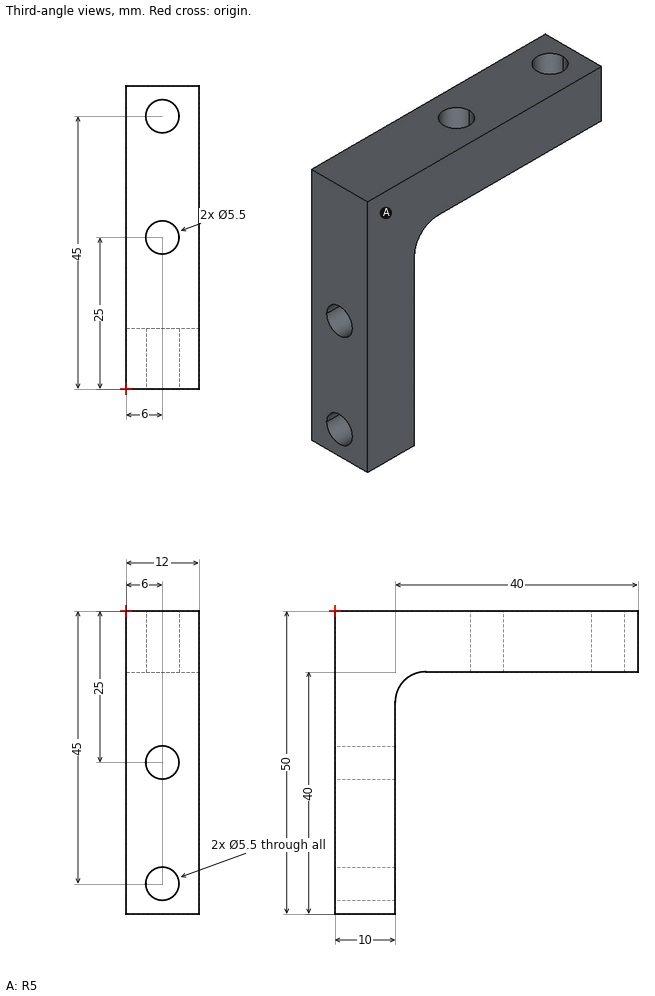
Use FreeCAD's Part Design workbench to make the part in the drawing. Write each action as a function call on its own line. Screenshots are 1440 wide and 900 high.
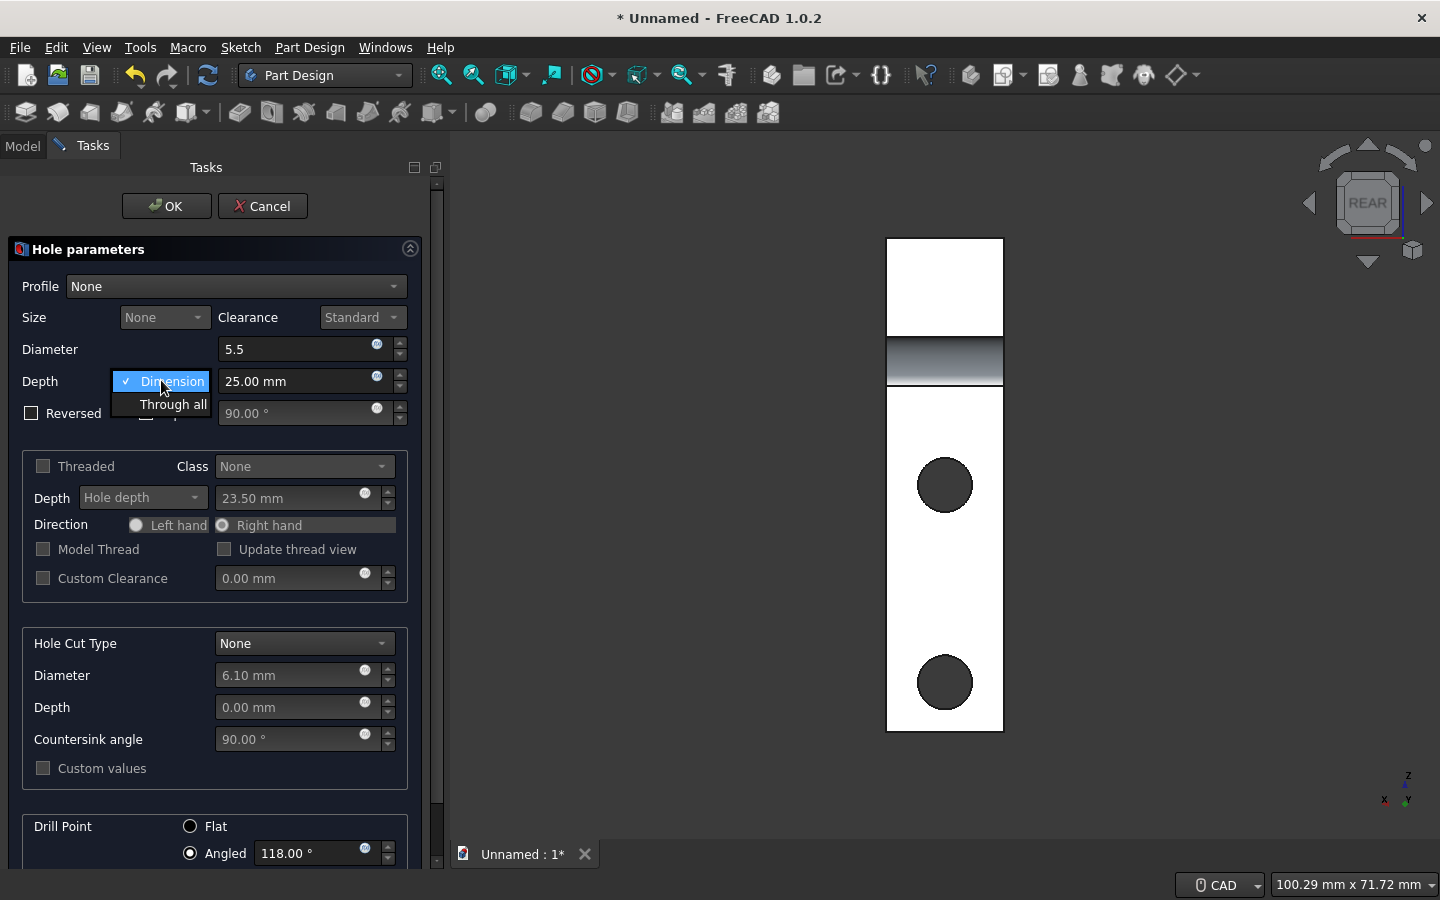
click(160, 404)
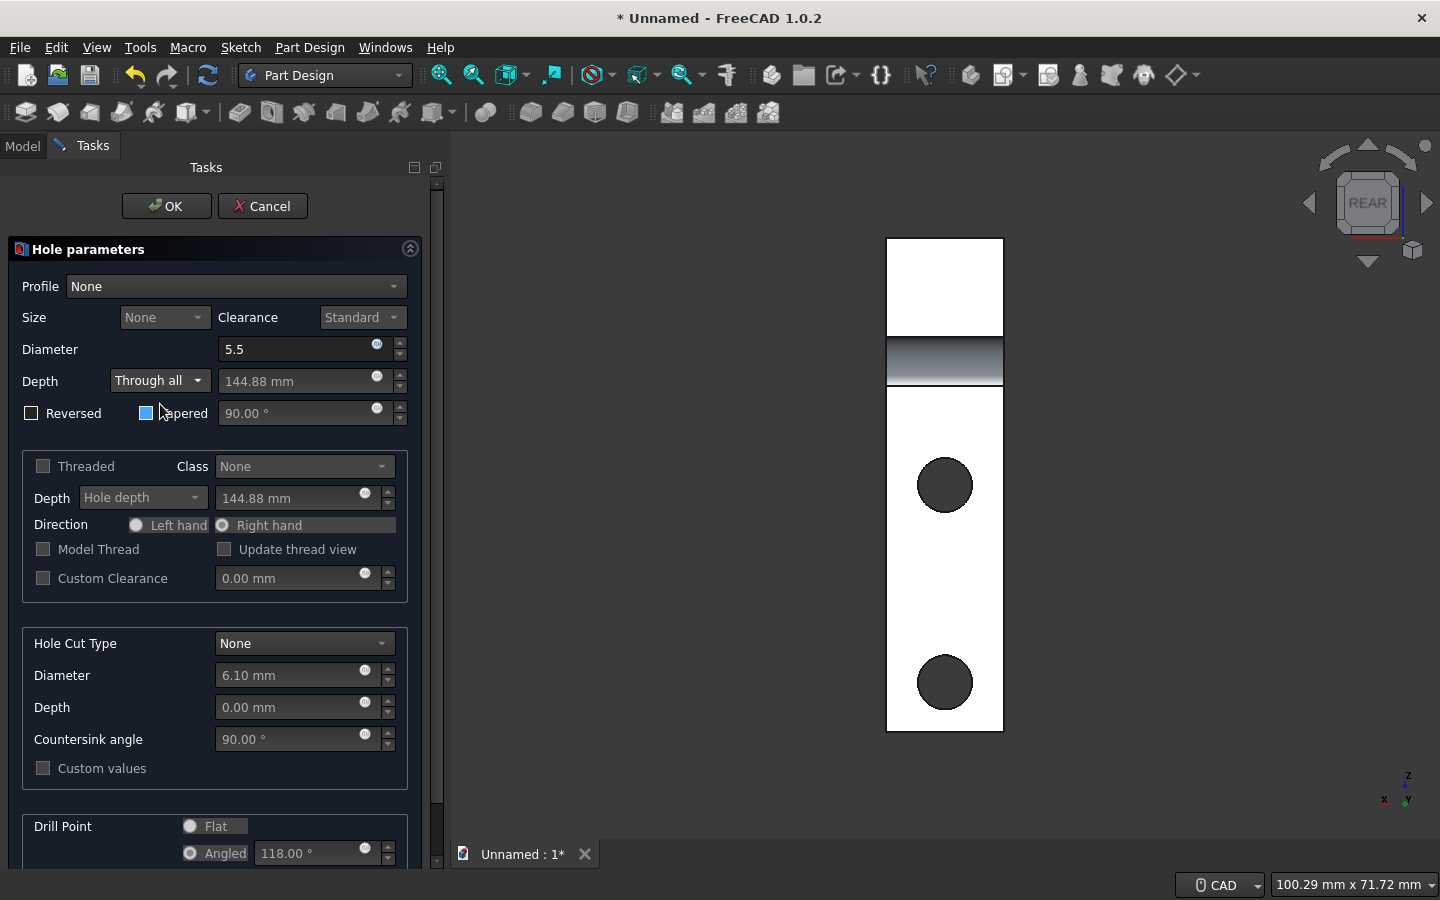
click(167, 206)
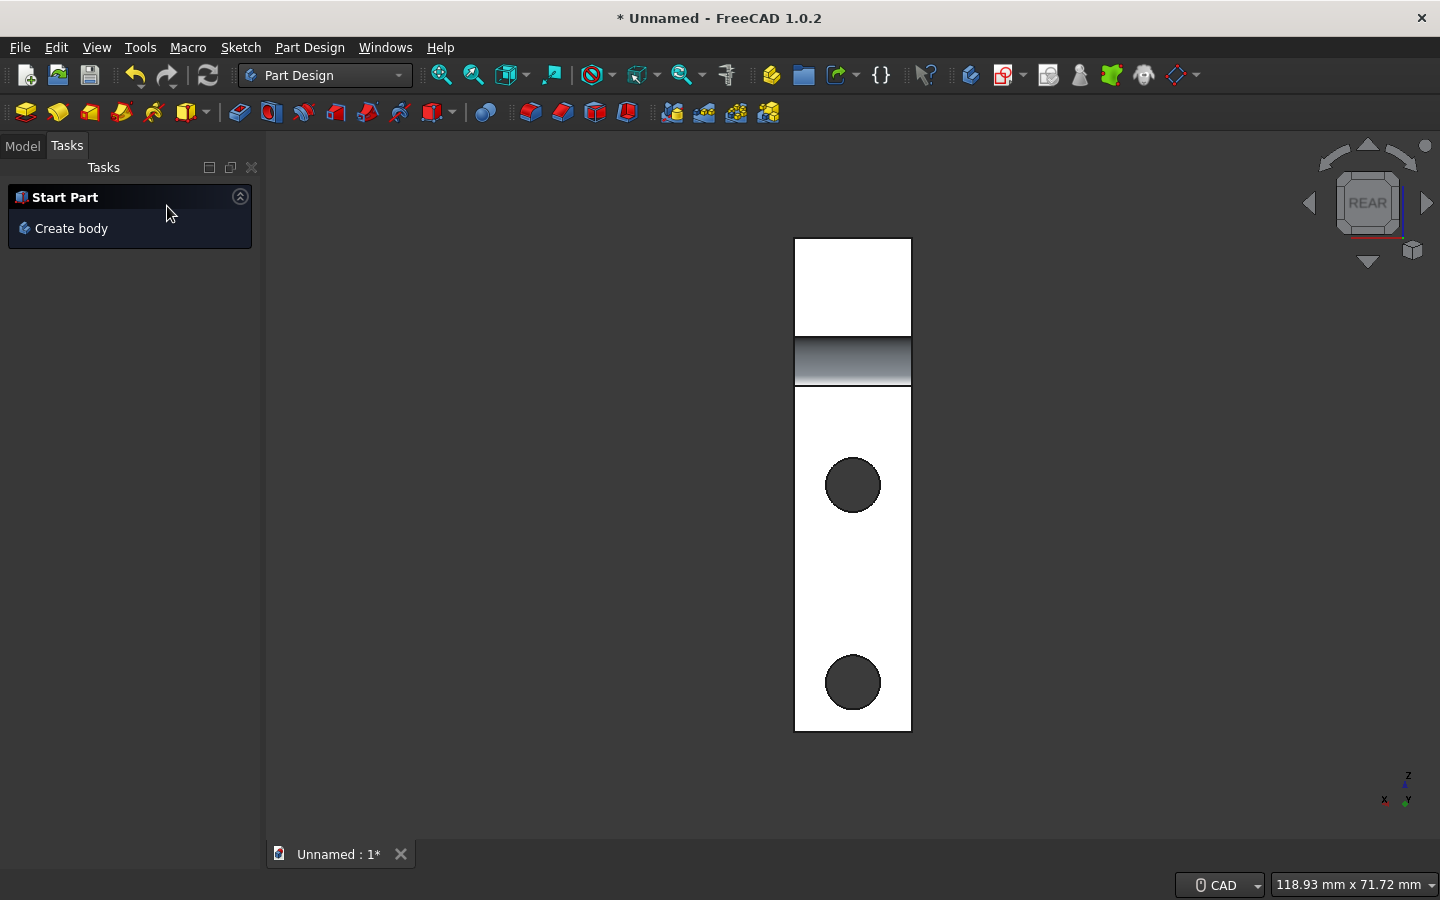
key(0)